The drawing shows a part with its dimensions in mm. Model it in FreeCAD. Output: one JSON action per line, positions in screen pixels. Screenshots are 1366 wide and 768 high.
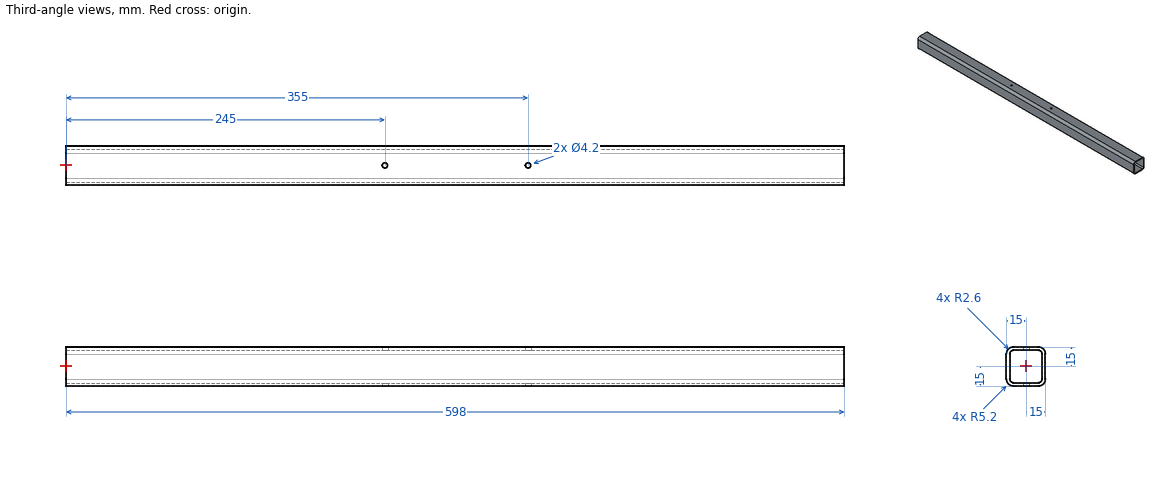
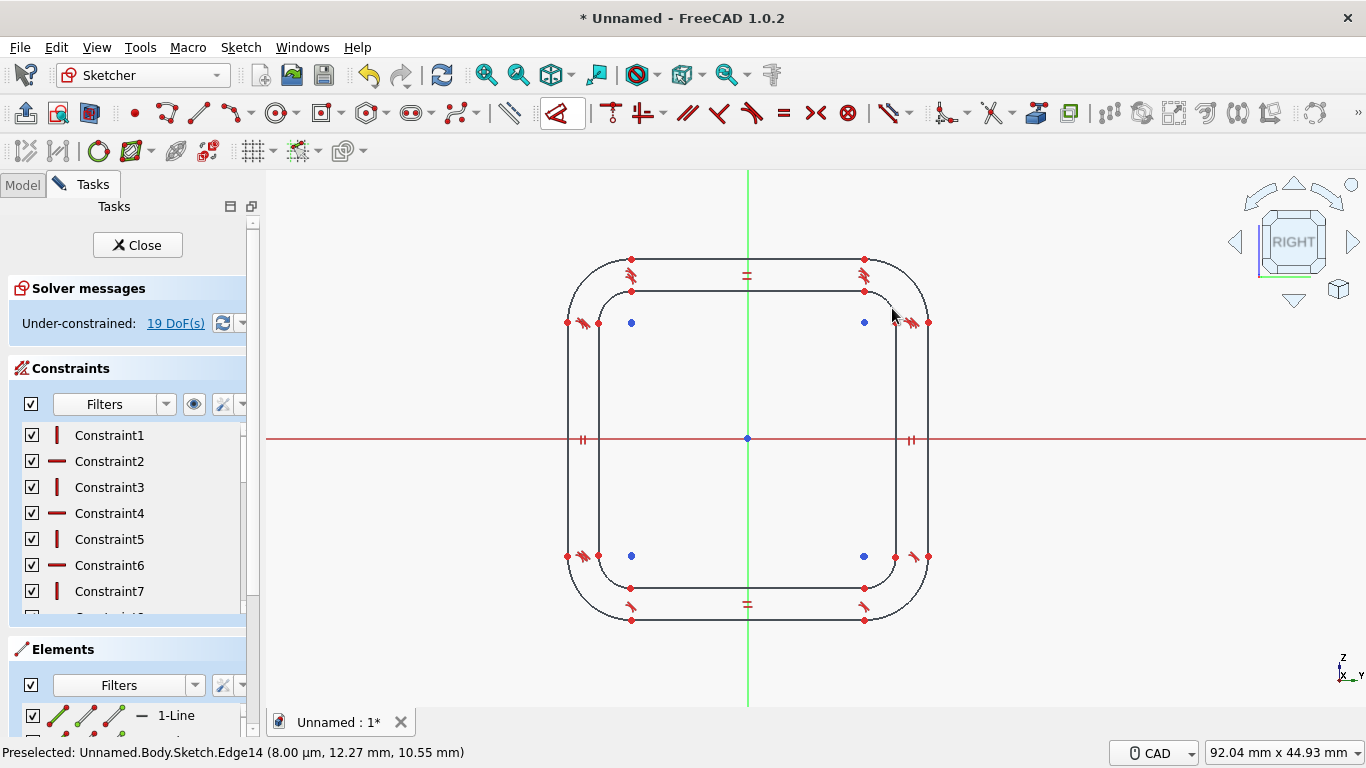
{"action": "left_click", "coordinate": [896, 393]}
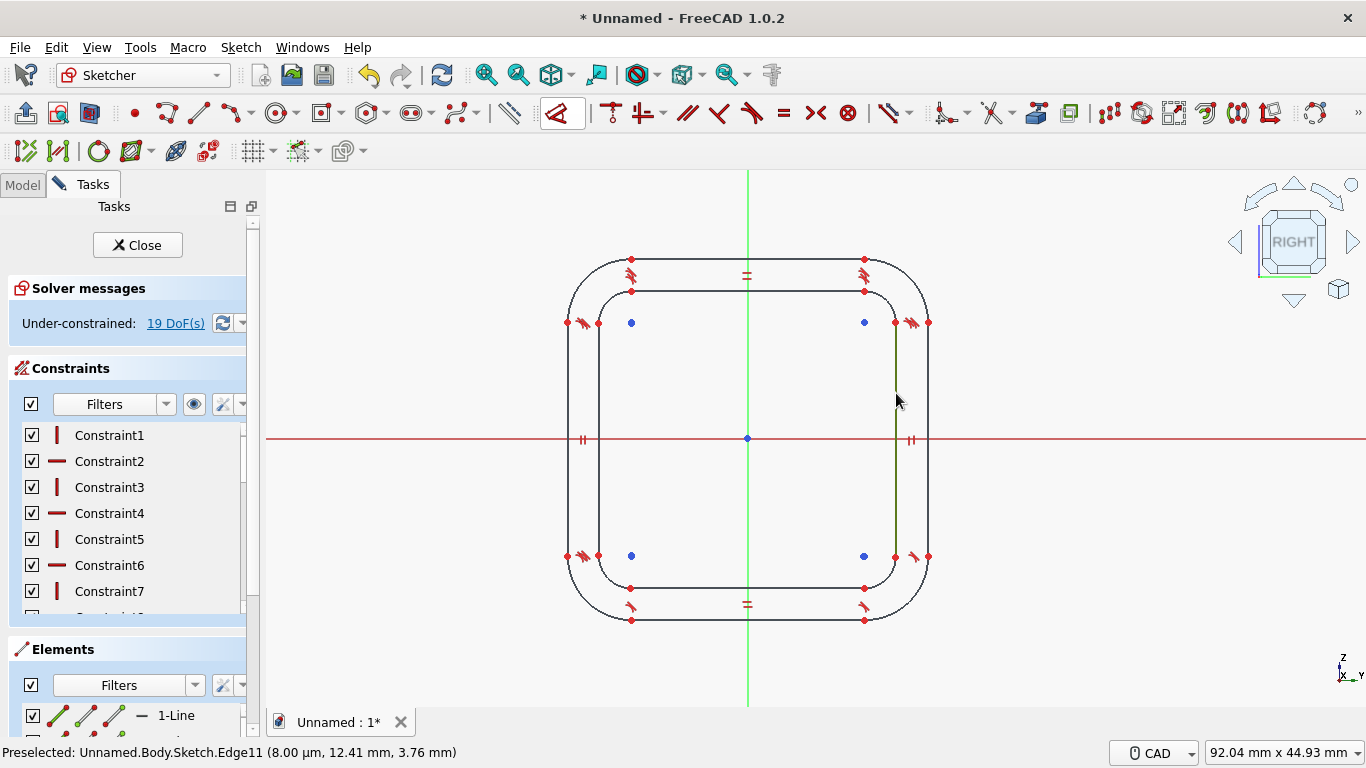
{"action": "left_click", "coordinate": [879, 585]}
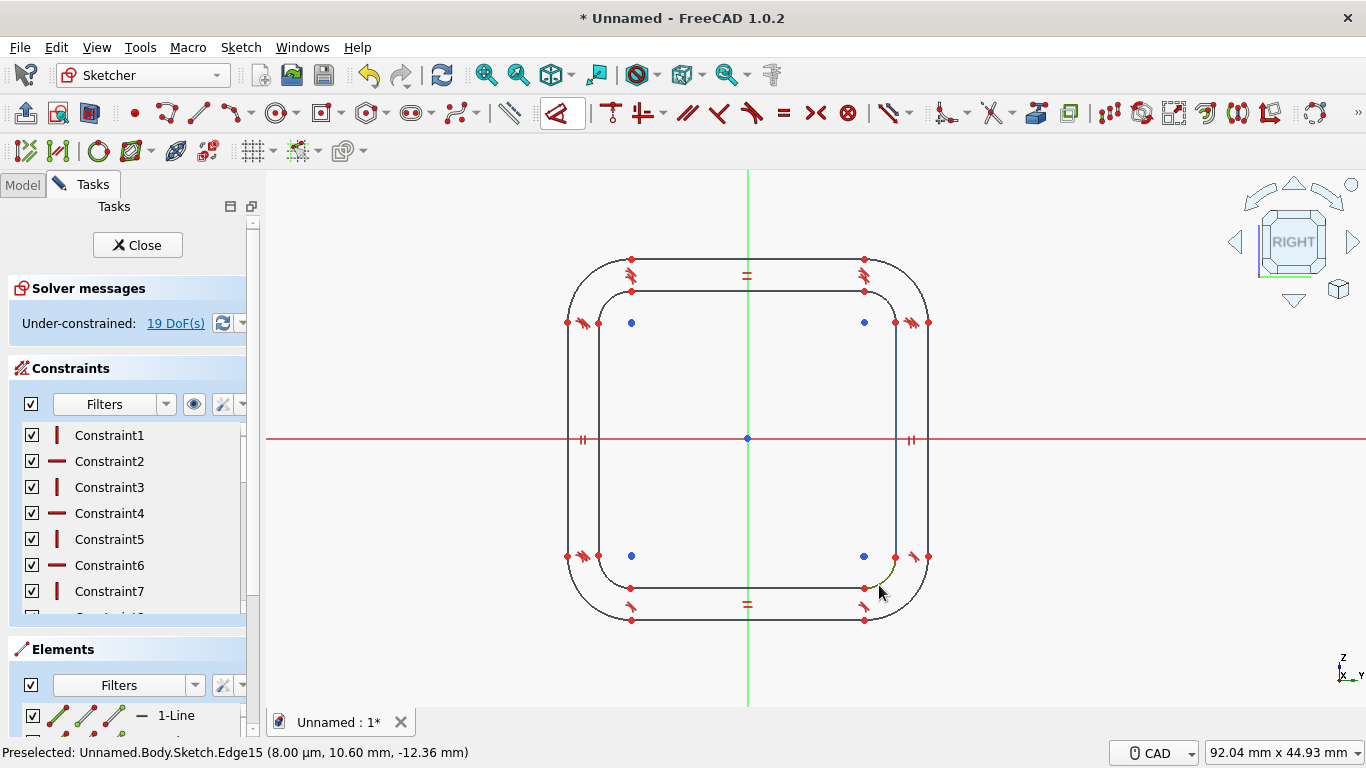
{"action": "left_click", "coordinate": [752, 114]}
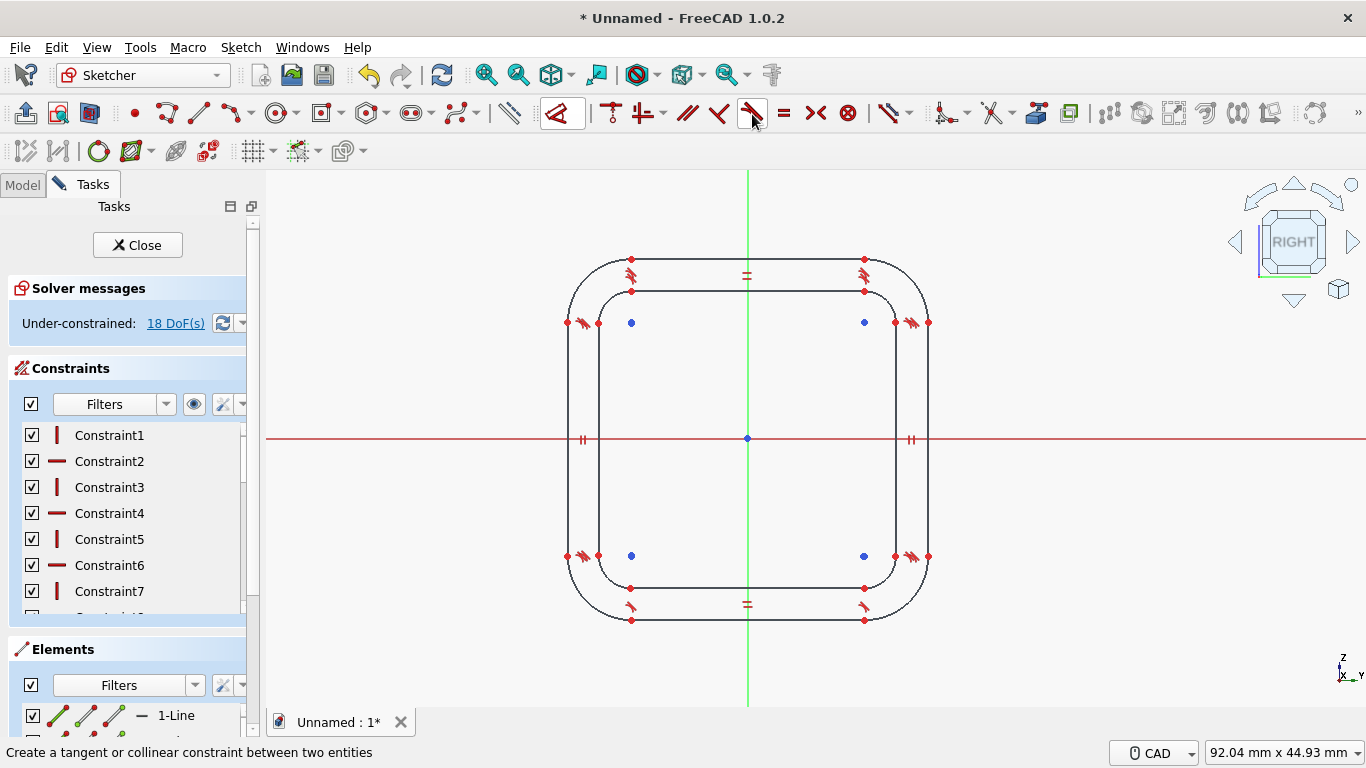
{"action": "left_click", "coordinate": [795, 588]}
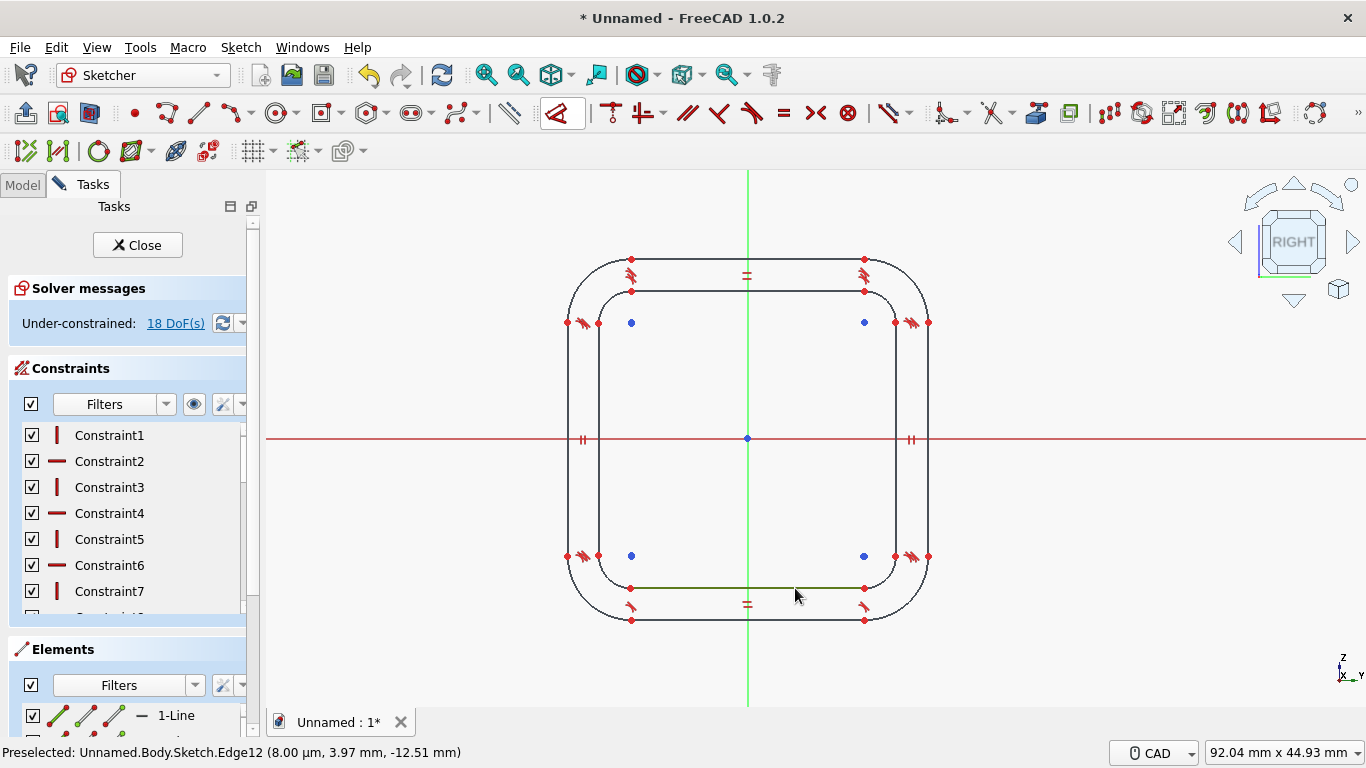
{"action": "left_click", "coordinate": [879, 585]}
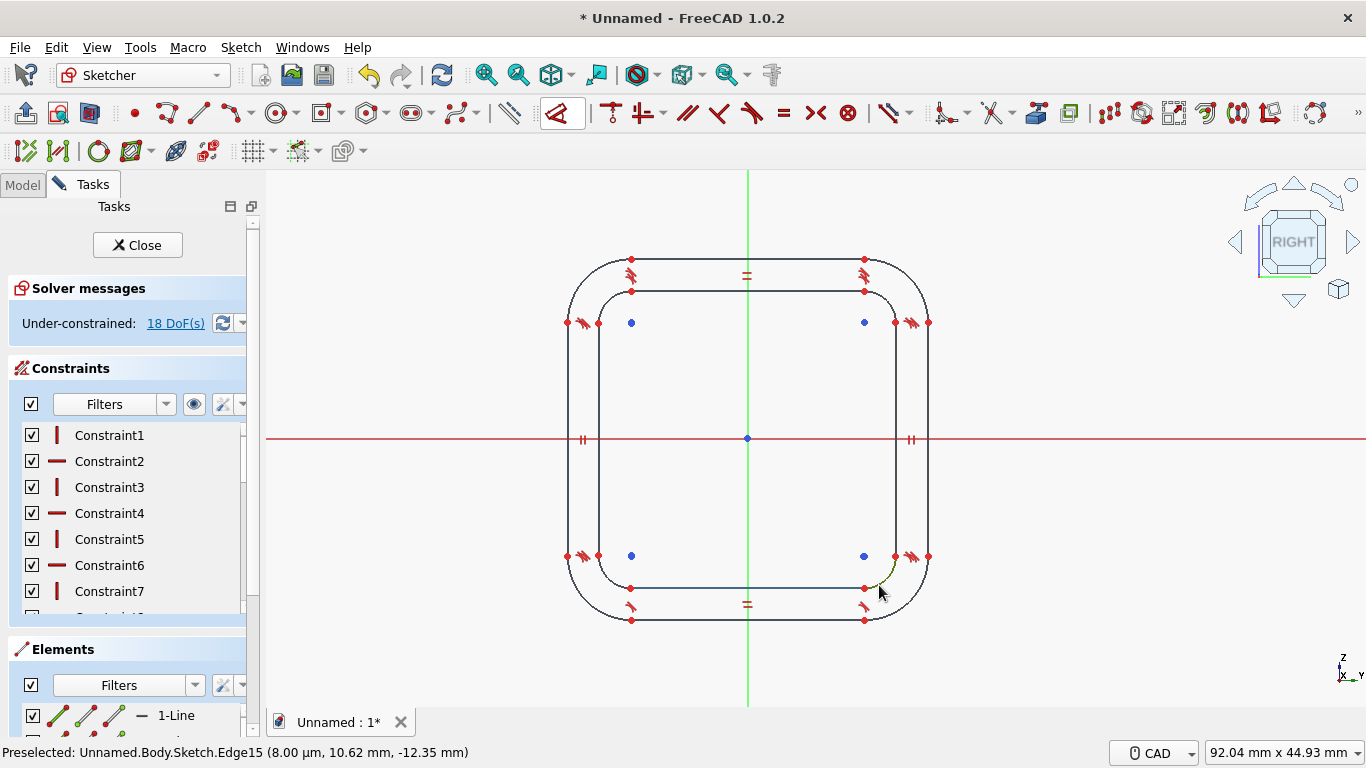
{"action": "key", "text": "t"}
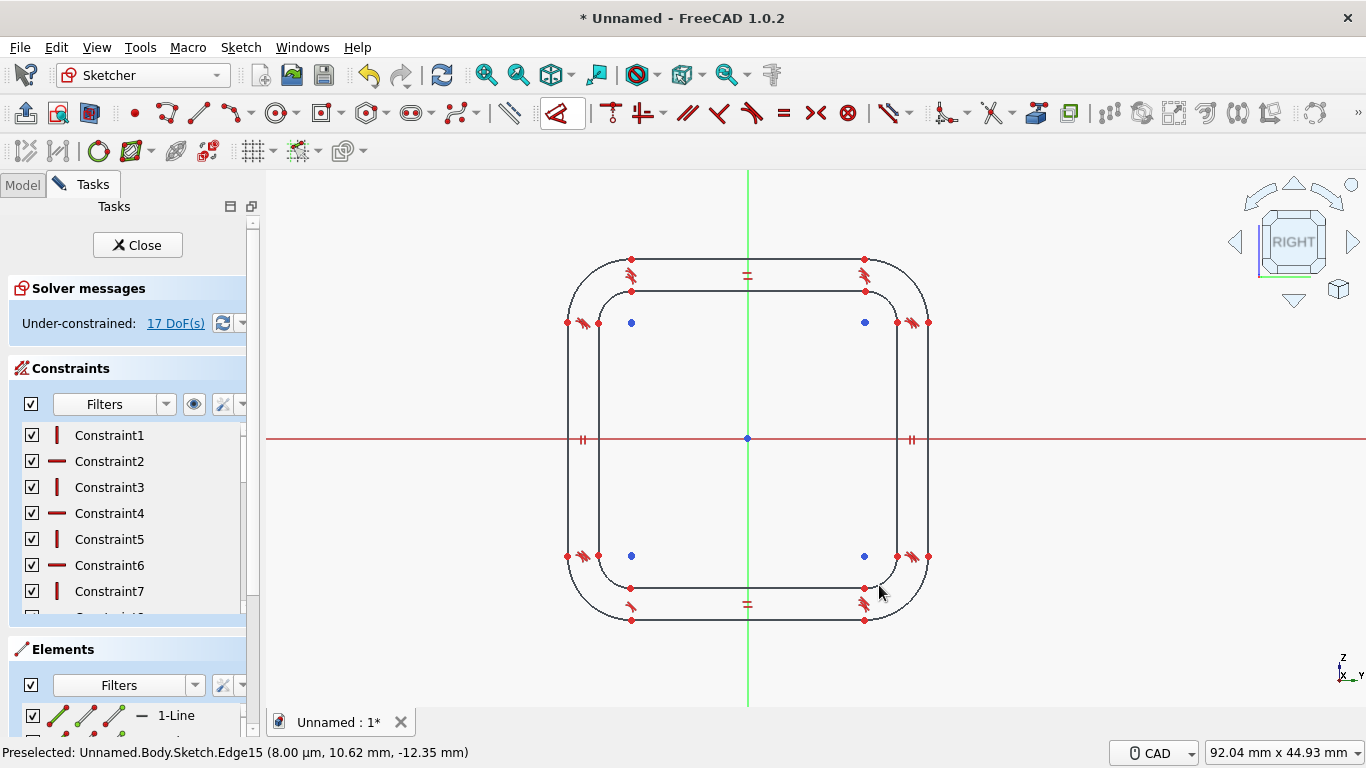
{"action": "left_click", "coordinate": [795, 588]}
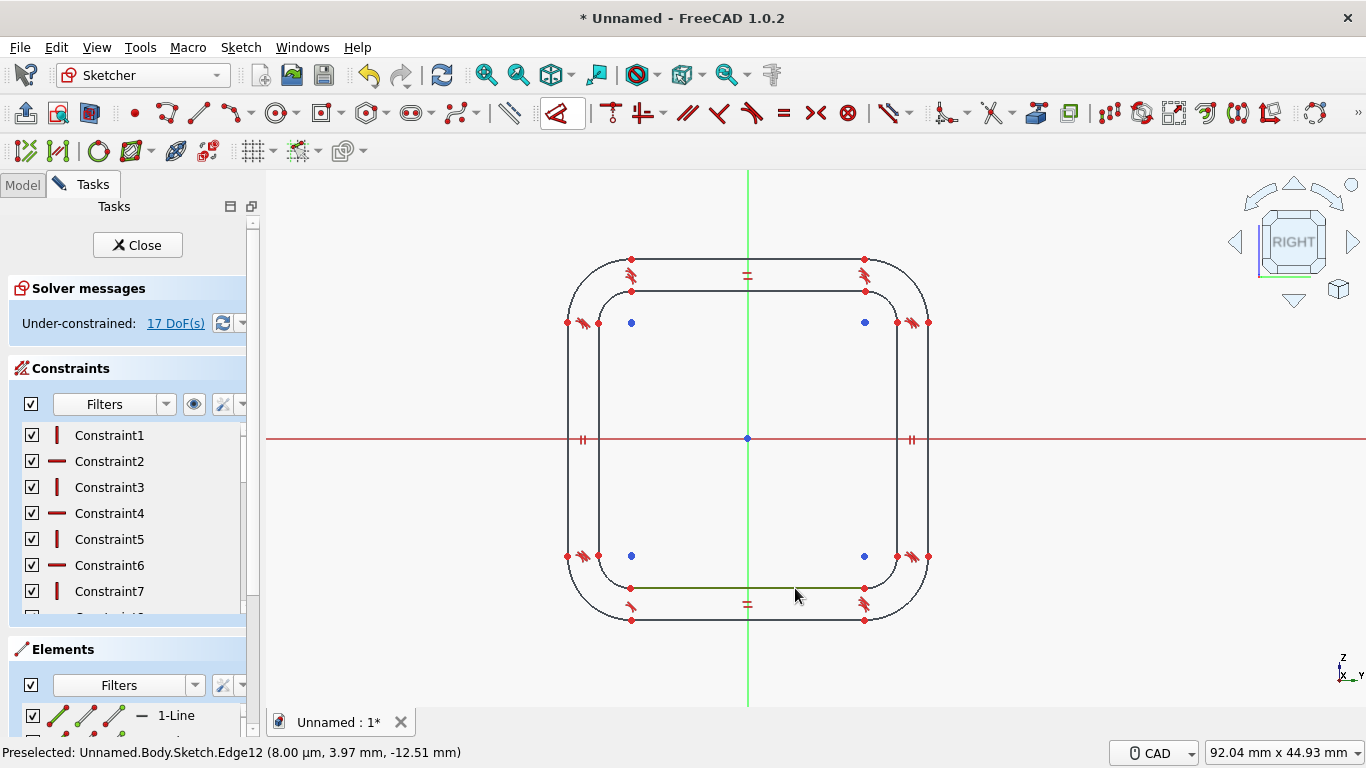
{"action": "left_click", "coordinate": [602, 570]}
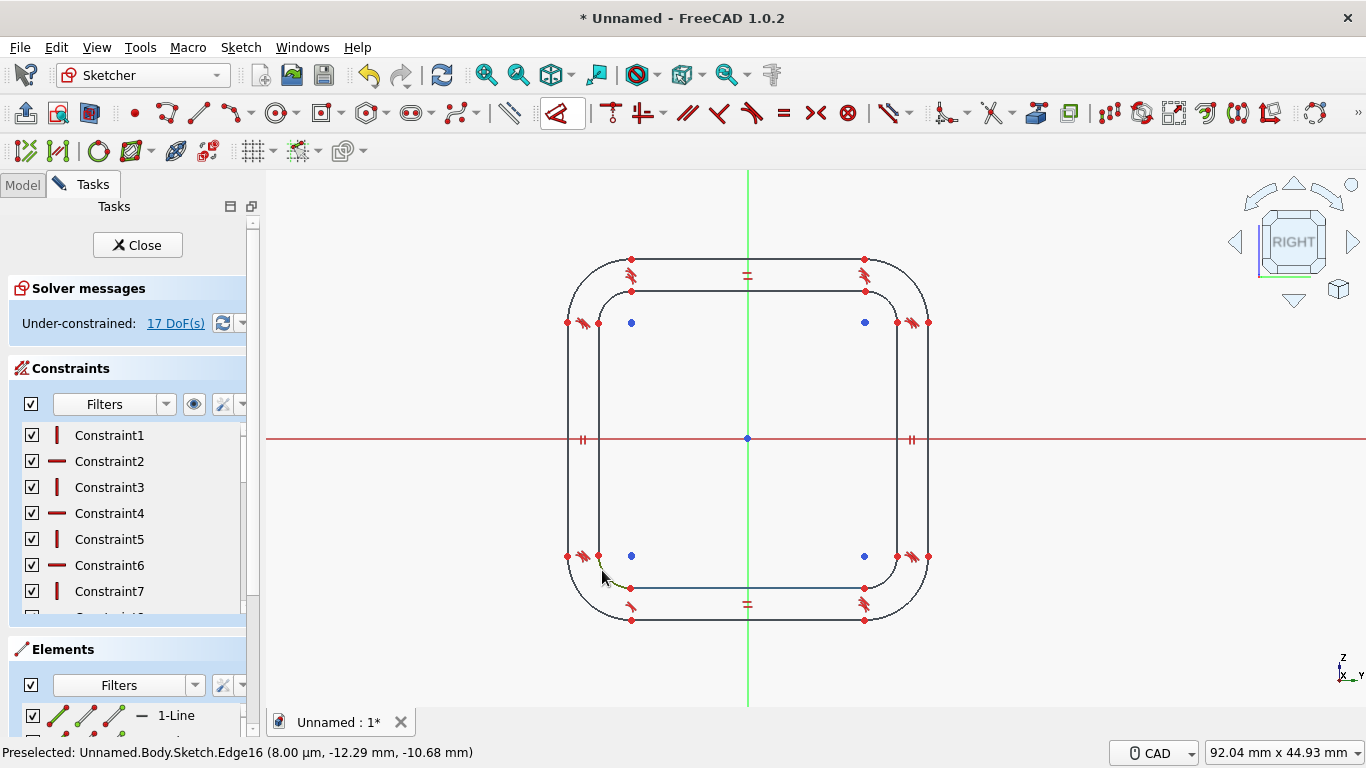
{"action": "key", "text": "t"}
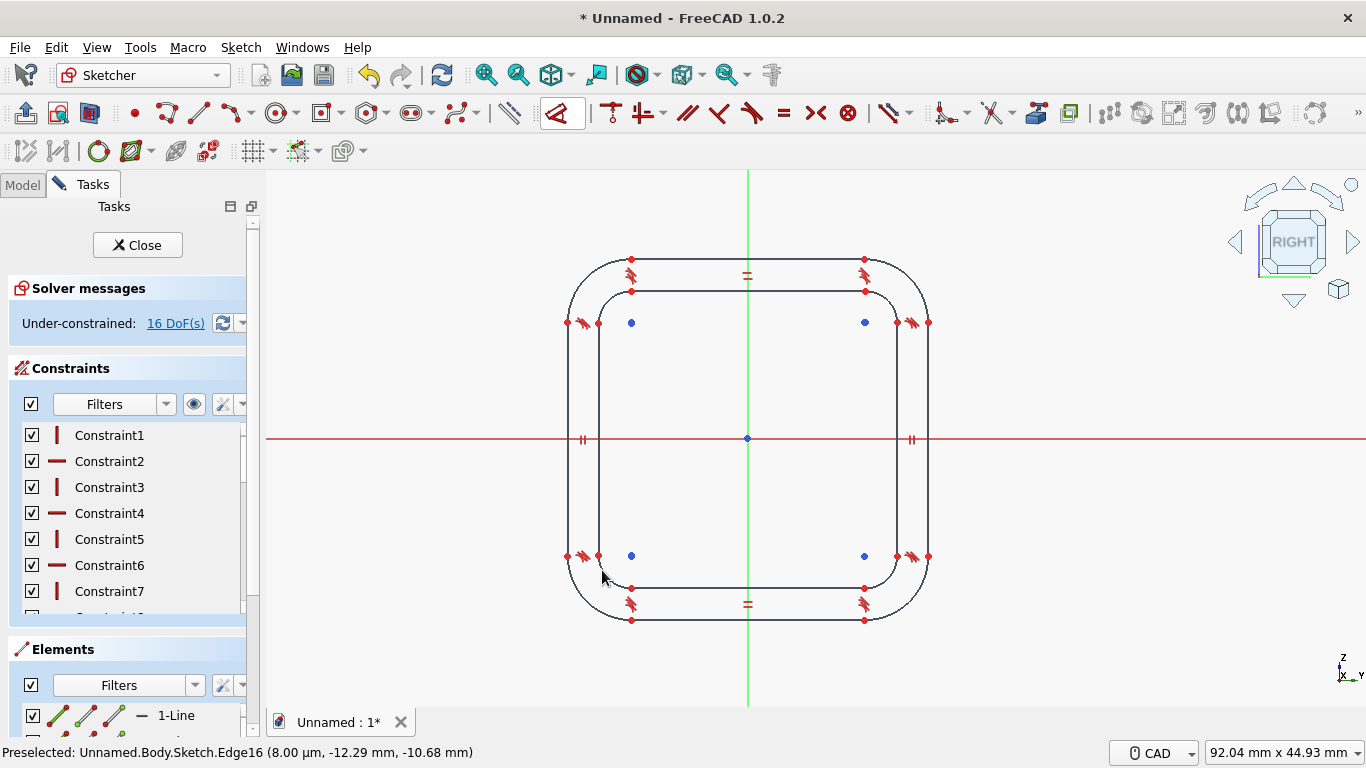
{"action": "left_click", "coordinate": [602, 266]}